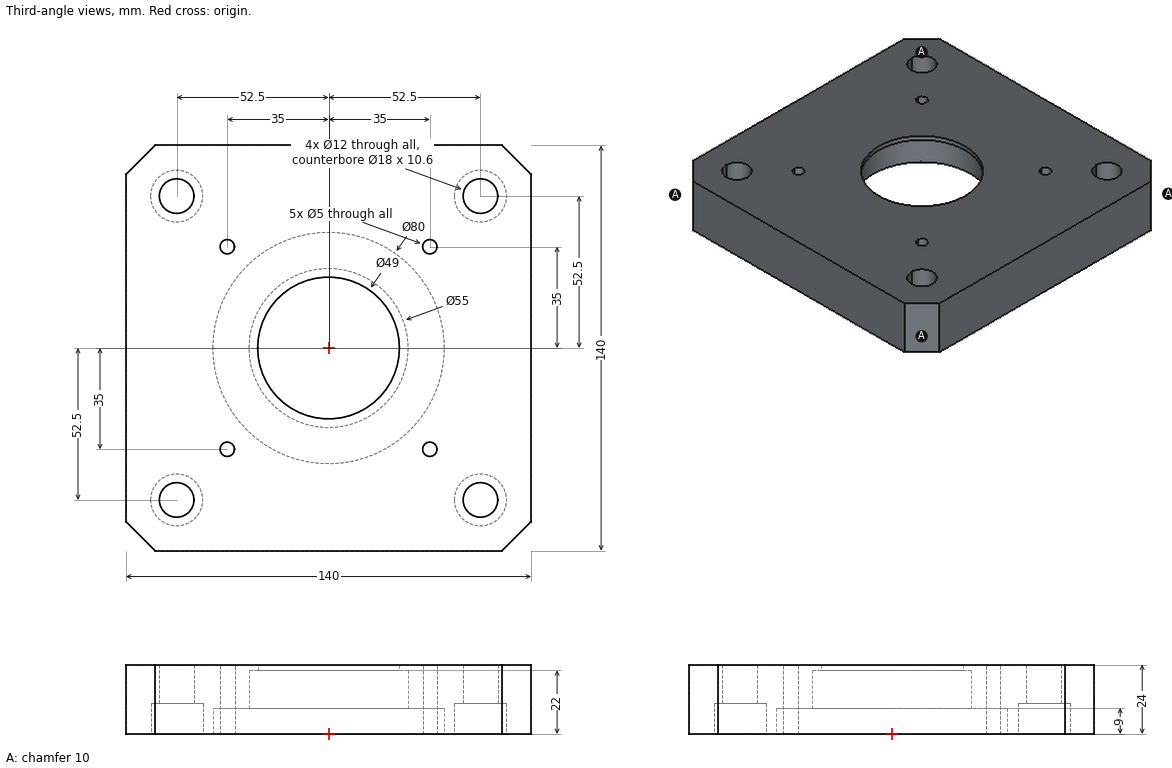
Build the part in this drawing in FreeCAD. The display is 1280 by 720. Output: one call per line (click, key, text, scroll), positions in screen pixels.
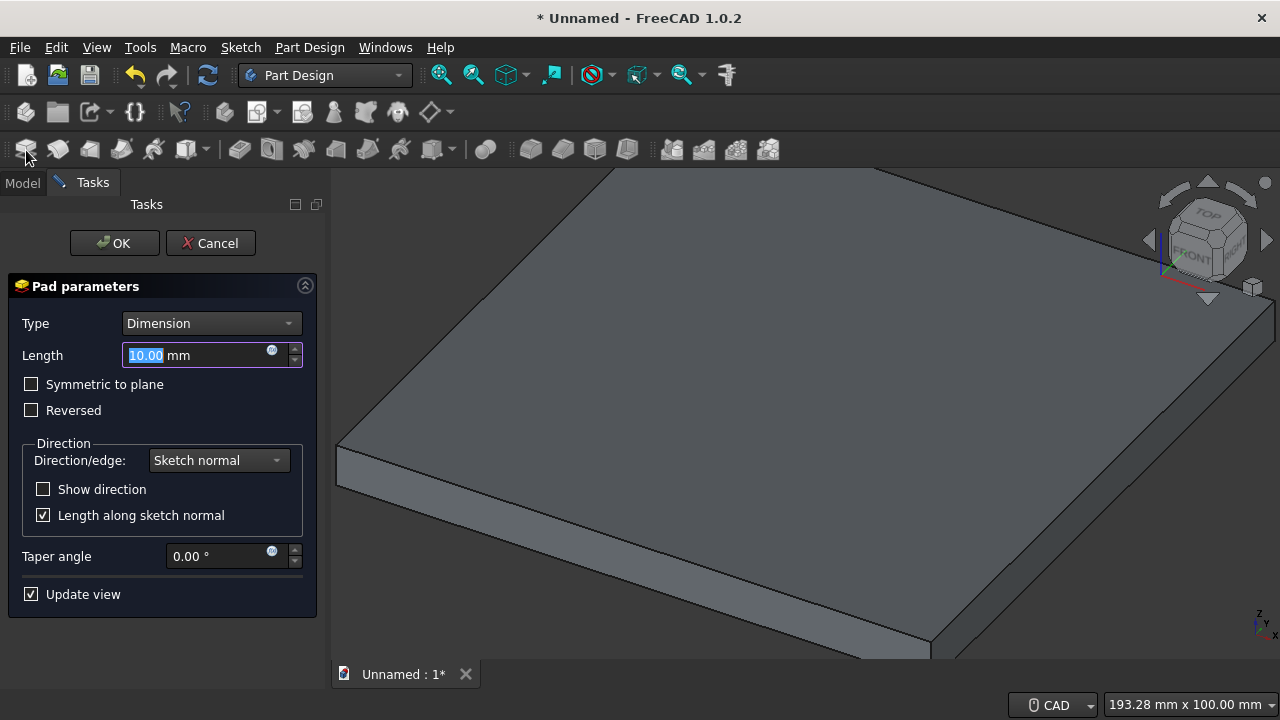
text(24)
key(Tab)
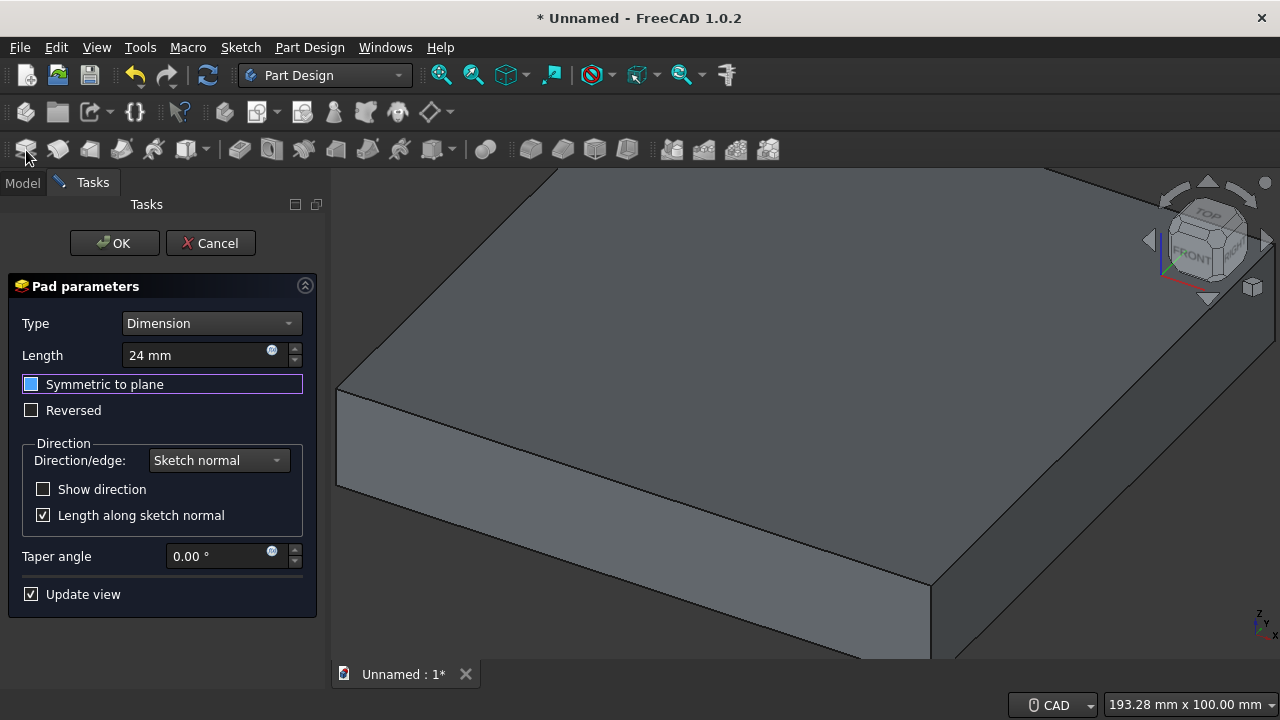
click(115, 243)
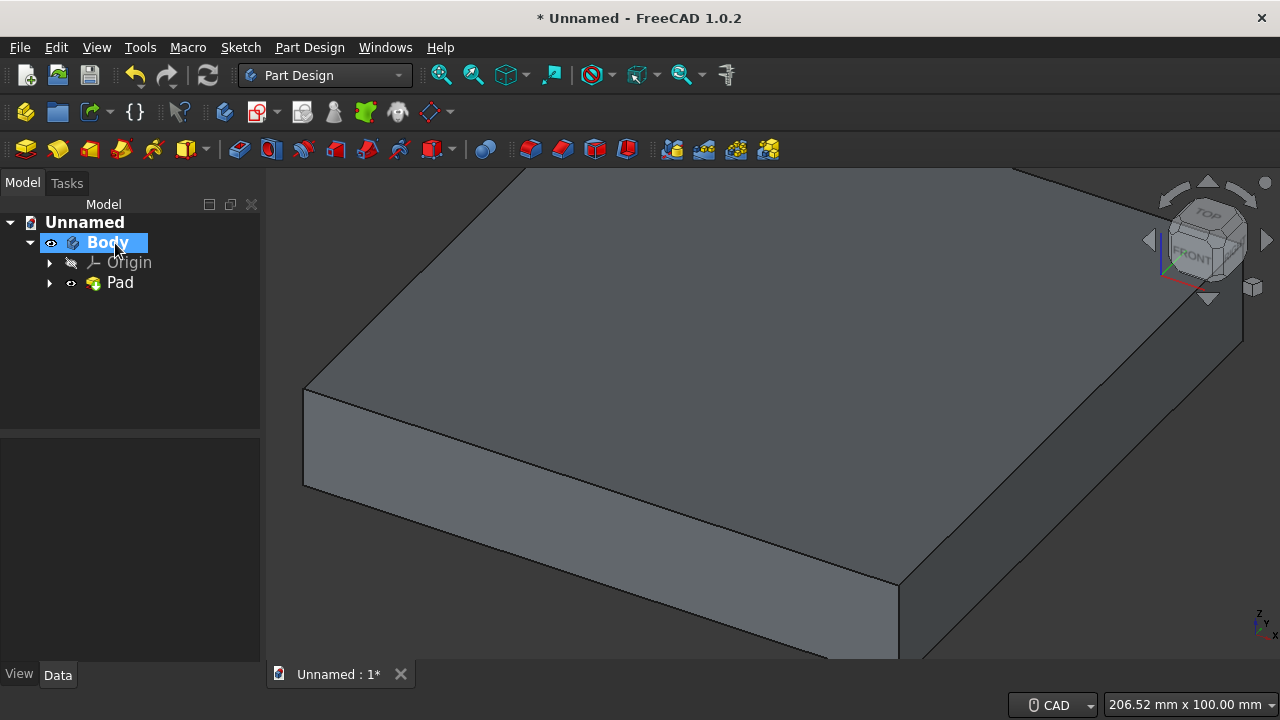
click(442, 76)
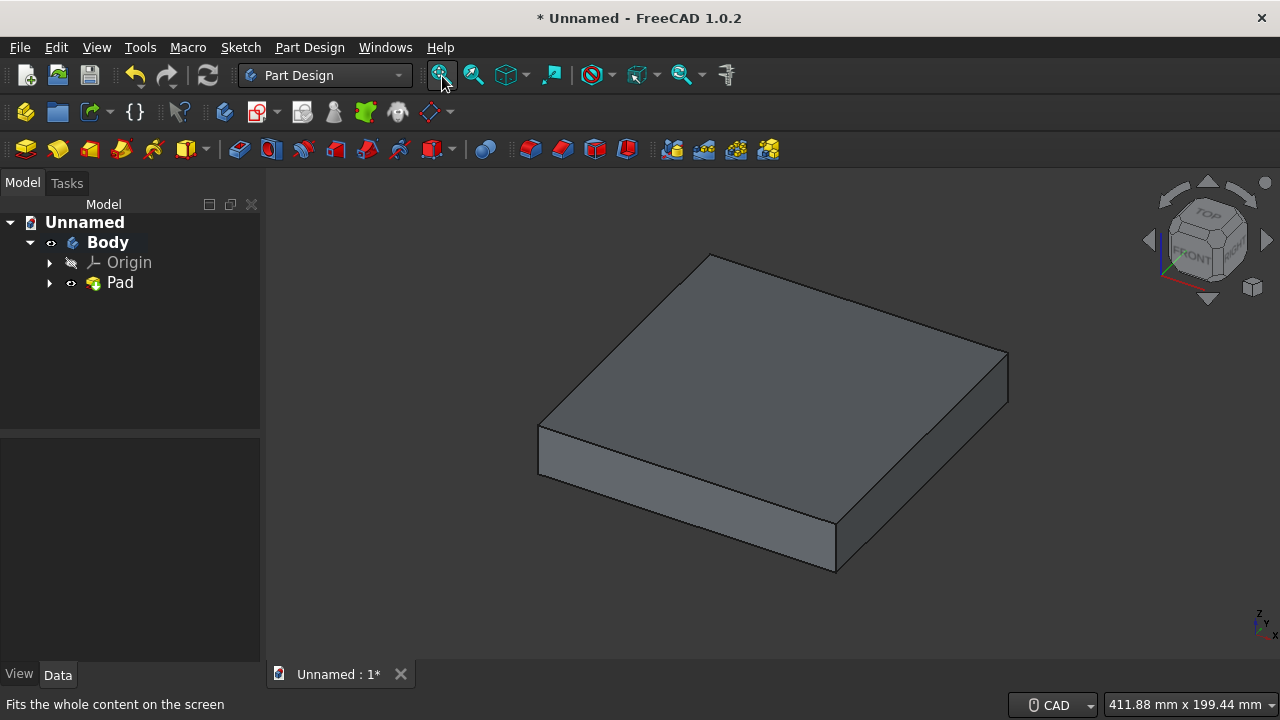
key(5)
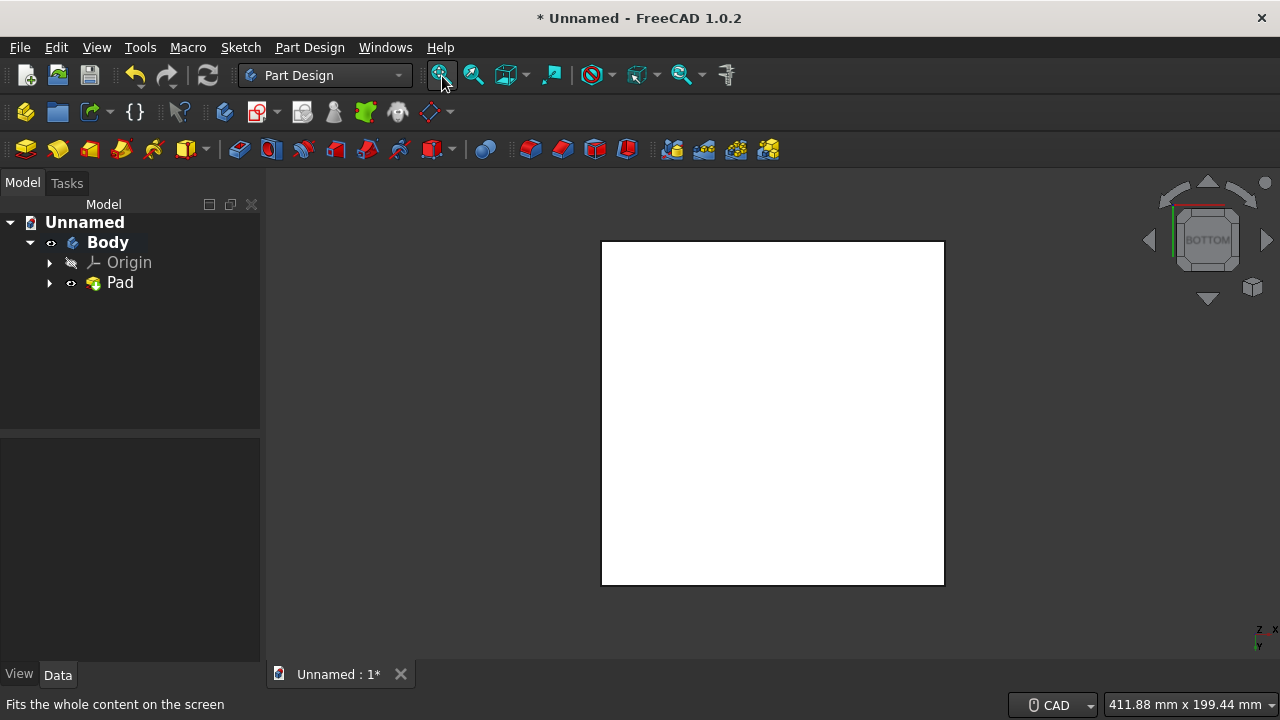
click(773, 412)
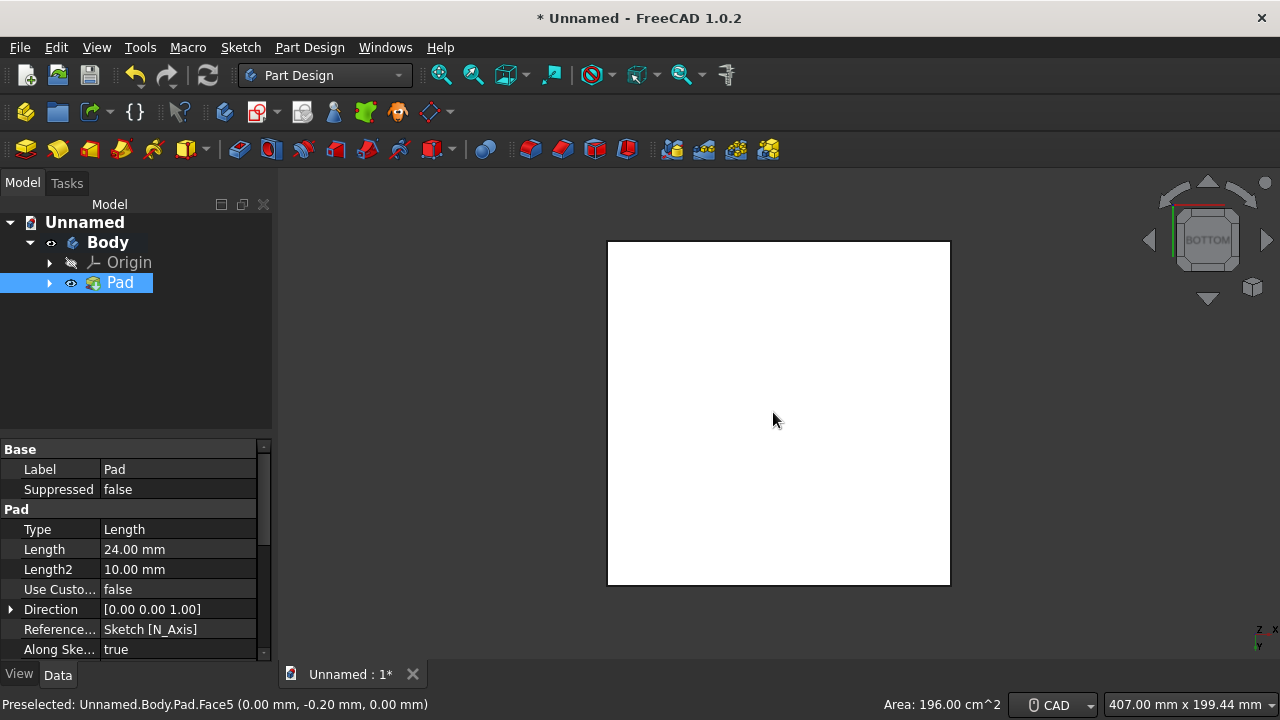
click(258, 112)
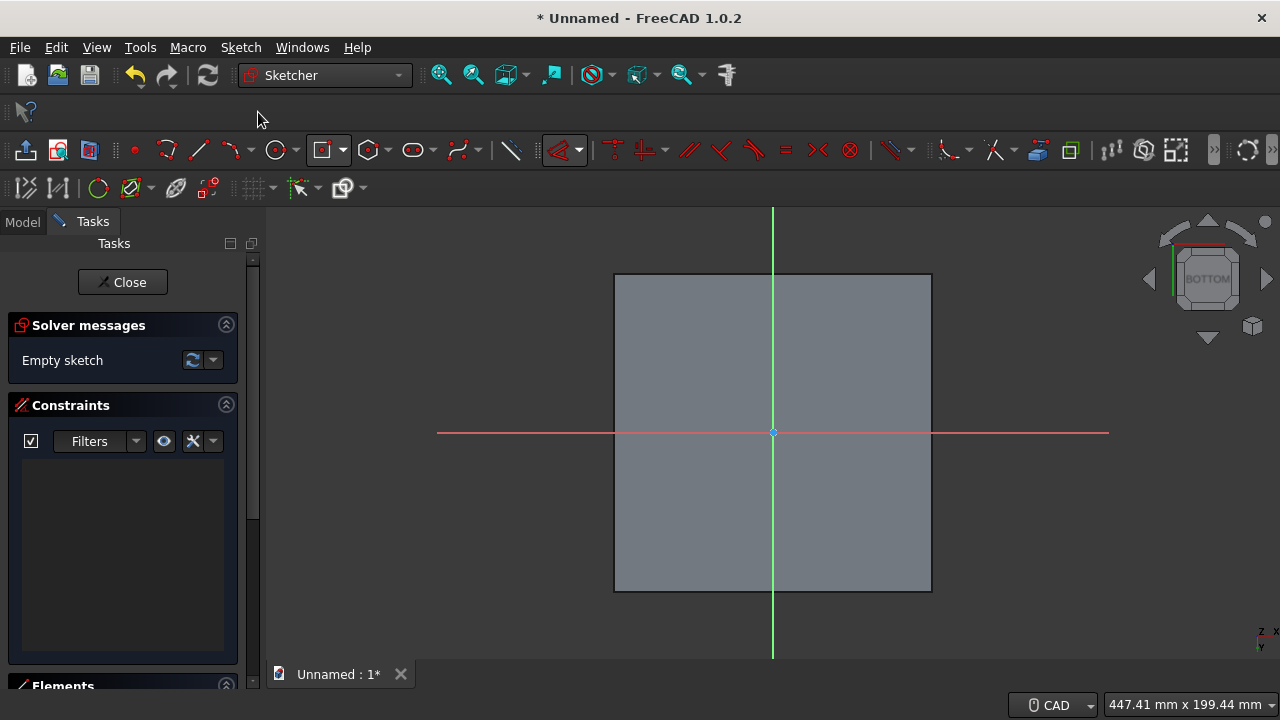
scroll(829, 433, up, 4)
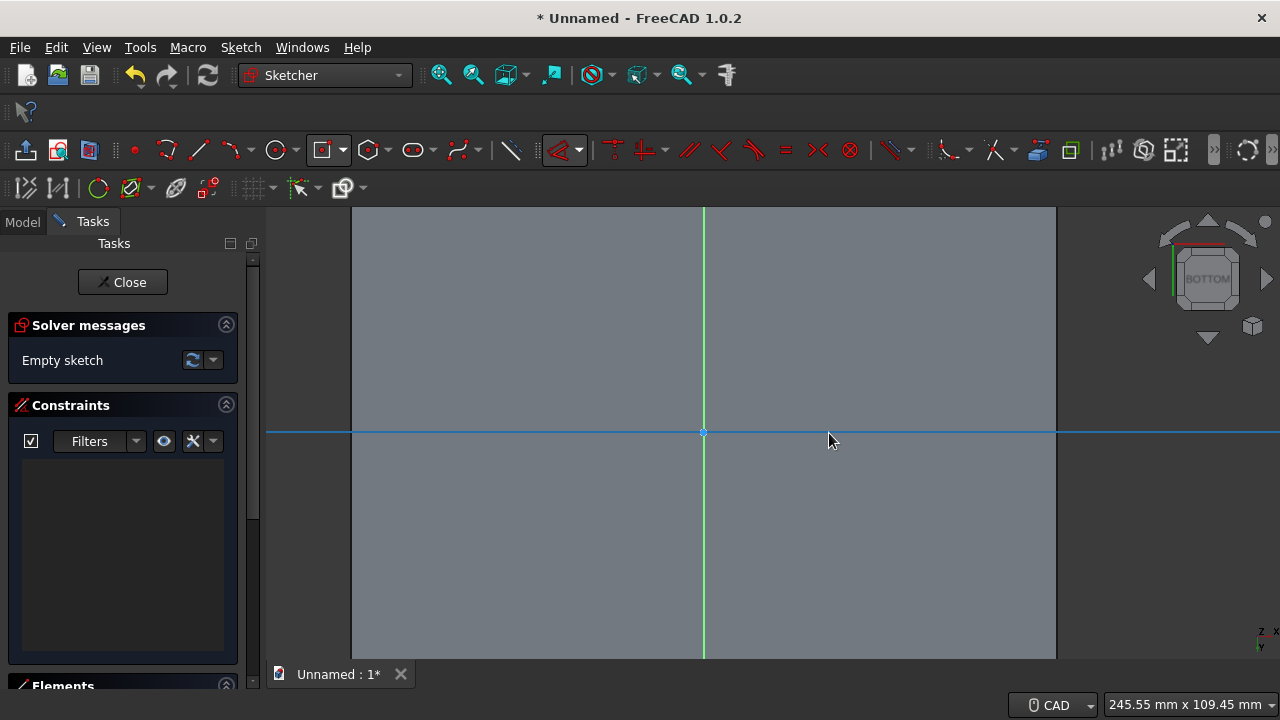
click(276, 150)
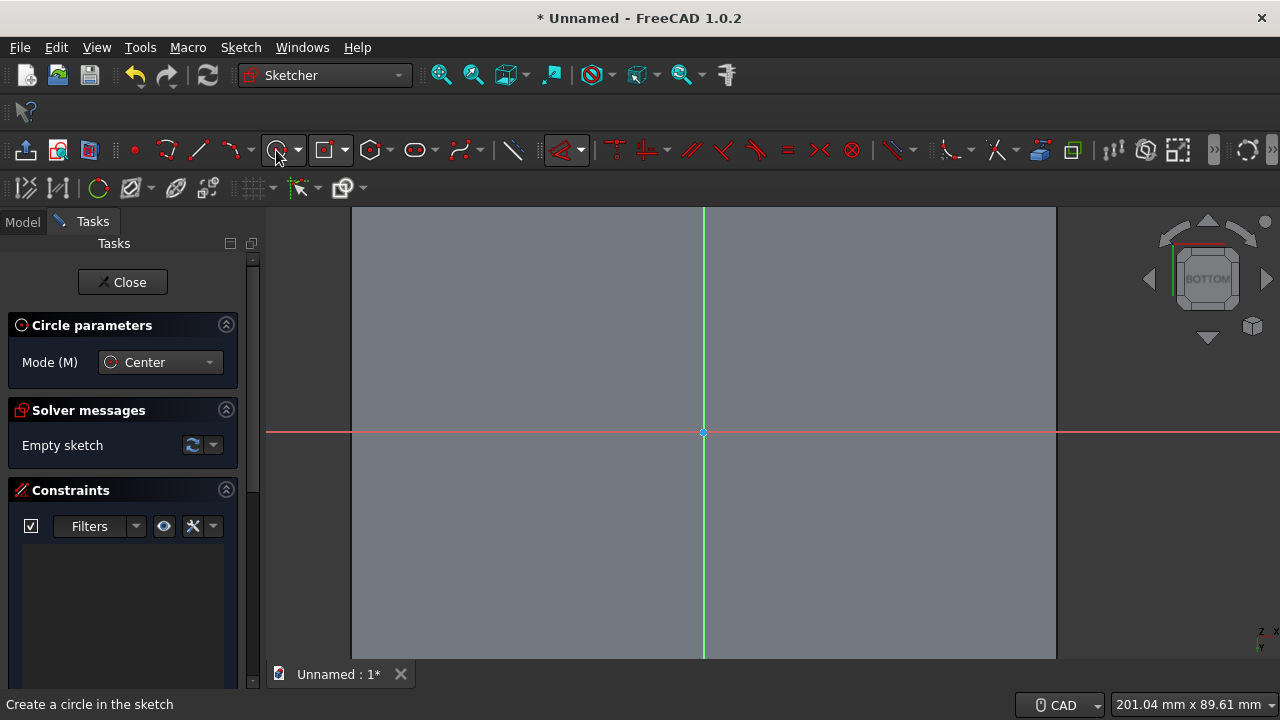
click(704, 432)
move(802, 334)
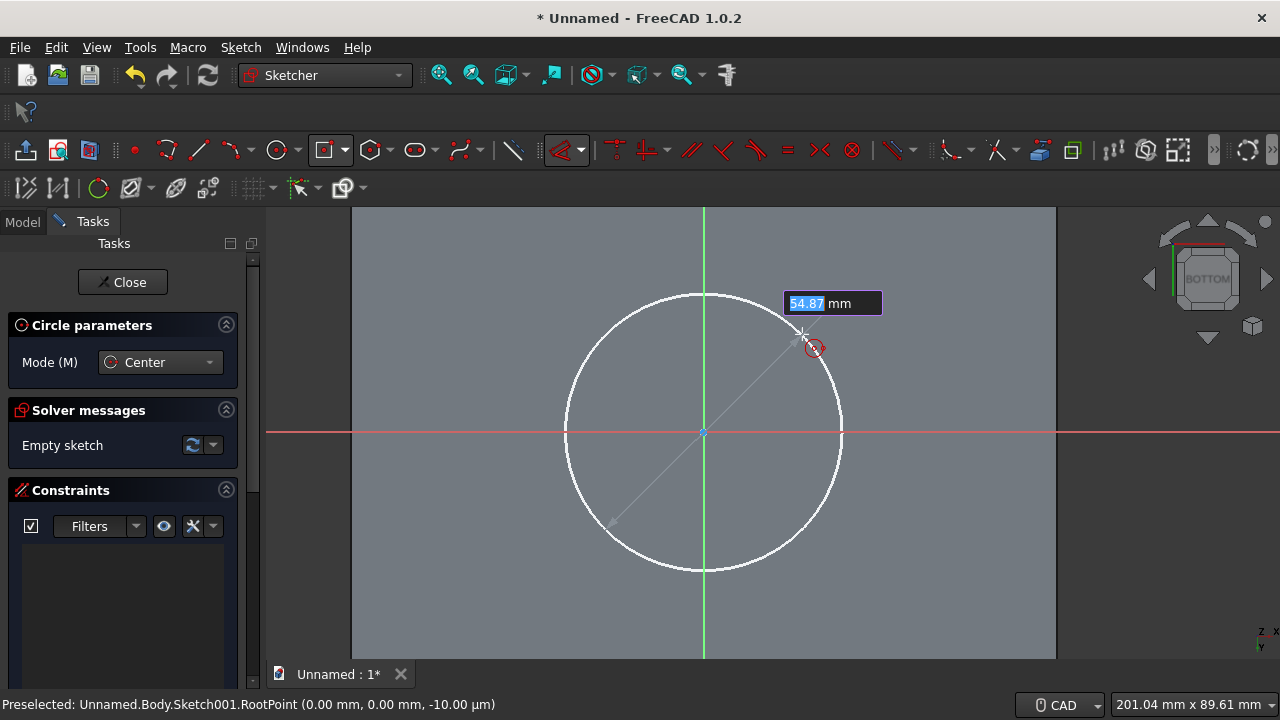
text(55)
key(Return)
key(Escape)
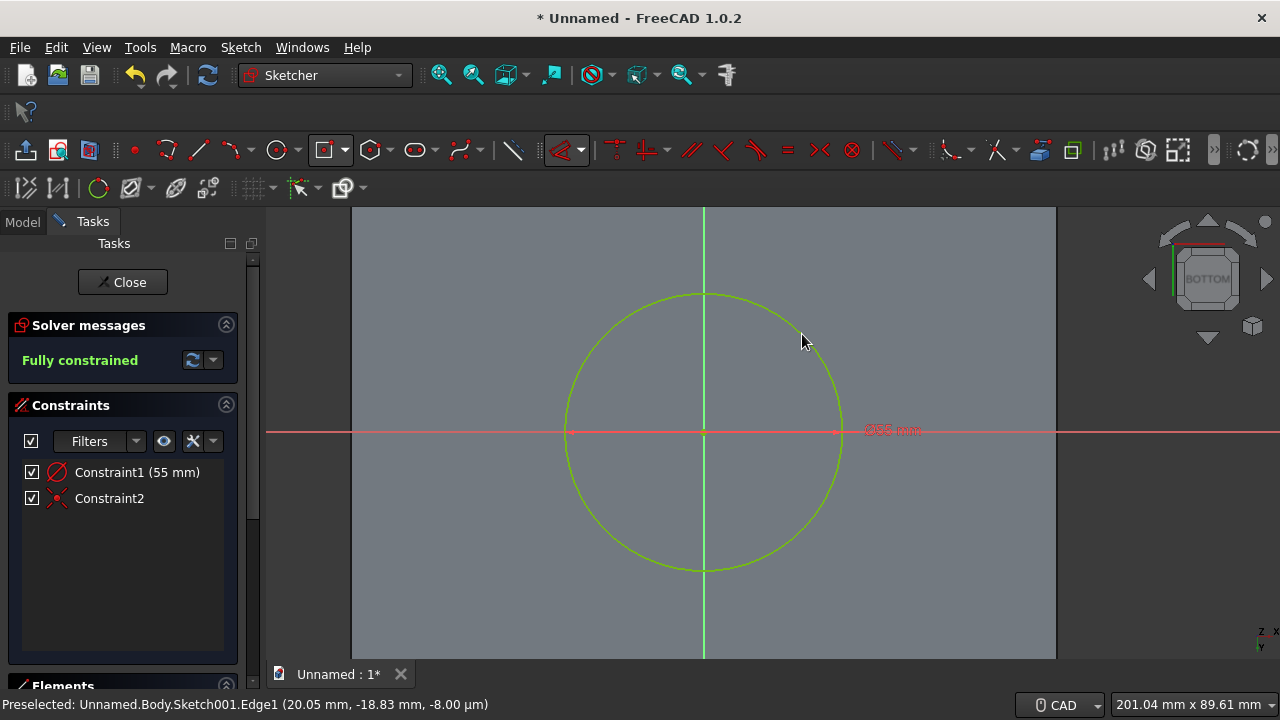
click(123, 282)